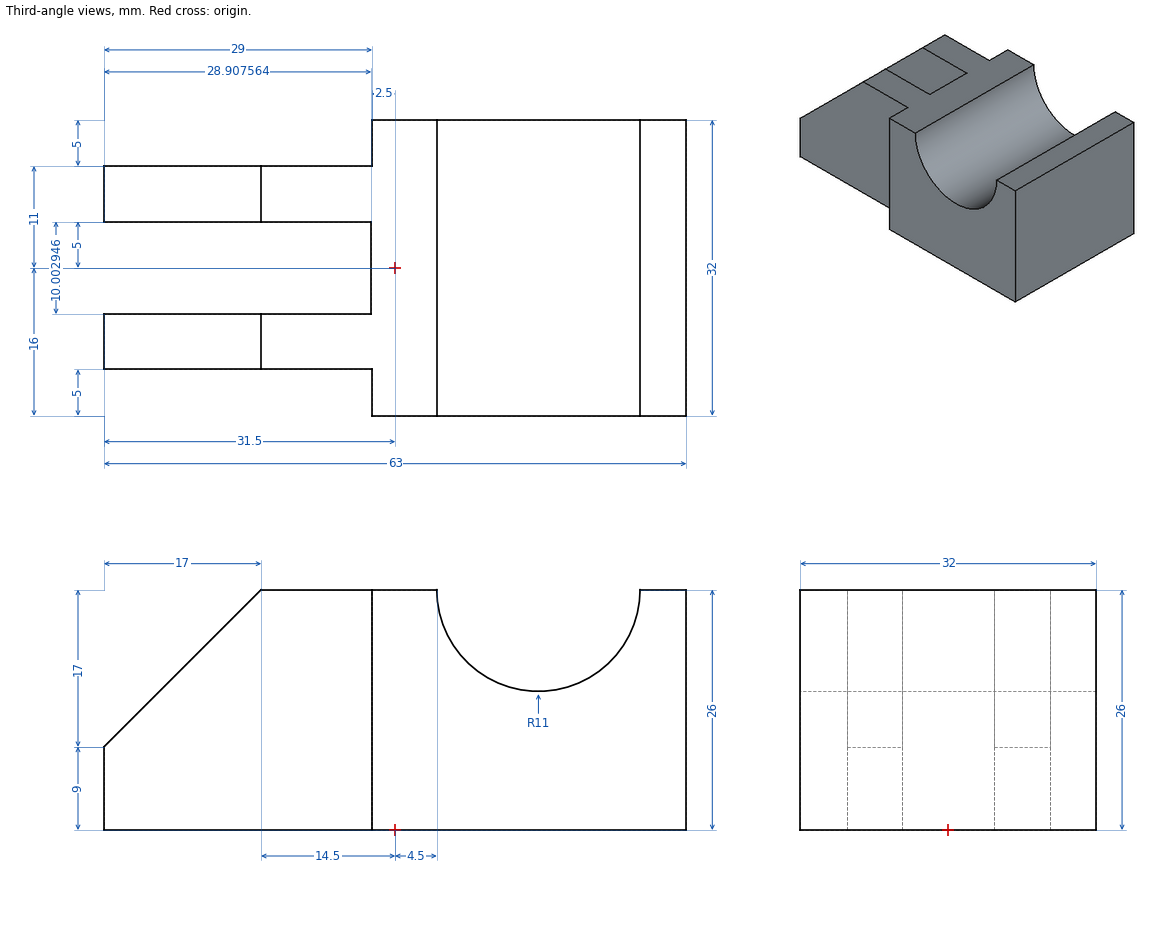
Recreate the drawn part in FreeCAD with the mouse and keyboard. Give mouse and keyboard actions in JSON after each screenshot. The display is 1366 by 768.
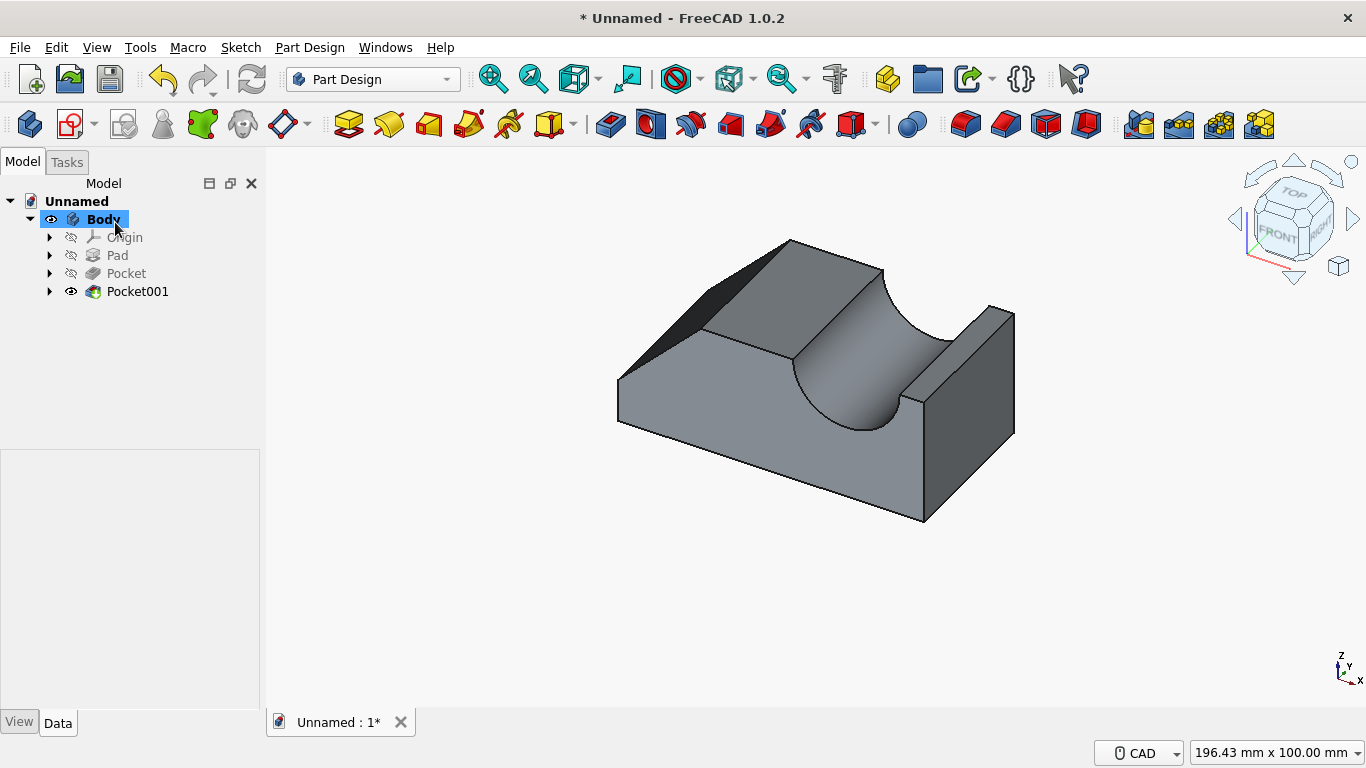
{"action": "key", "text": "5"}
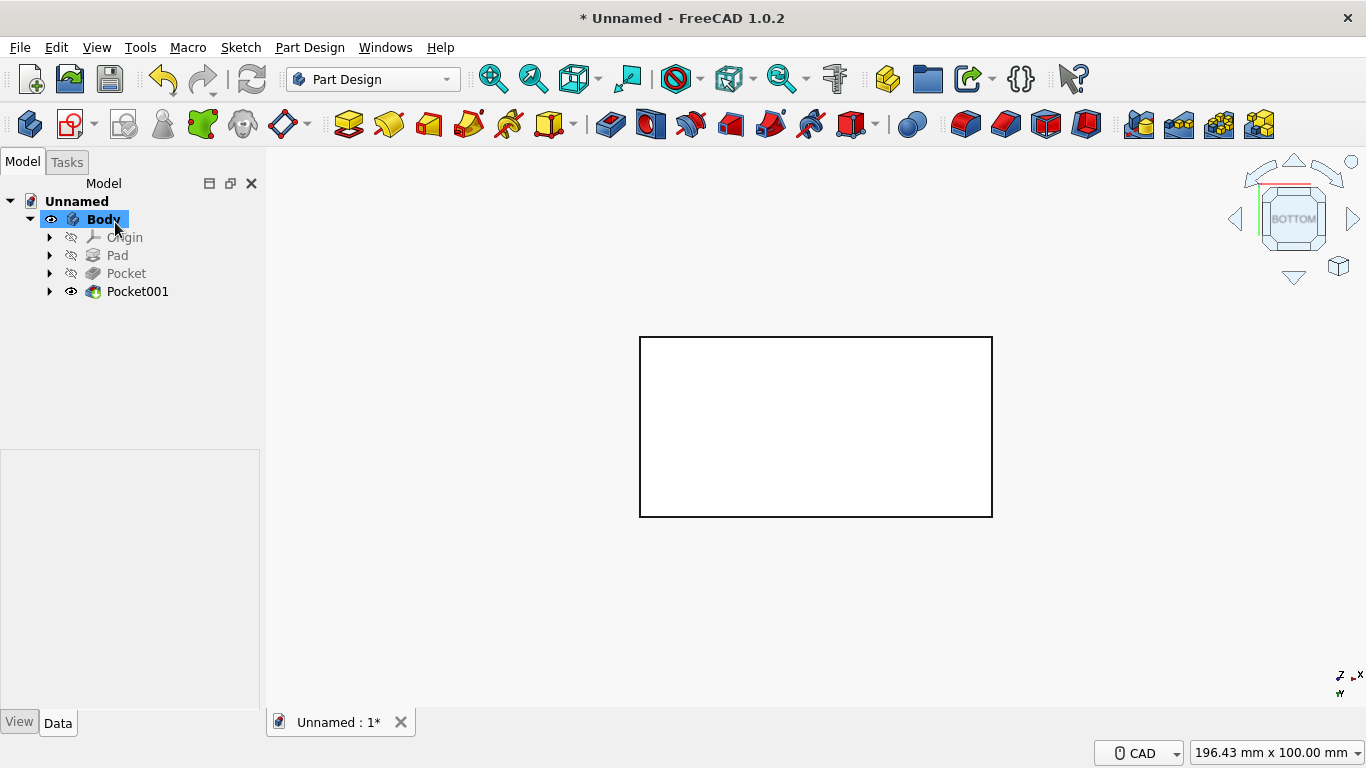
{"action": "left_click", "coordinate": [494, 80]}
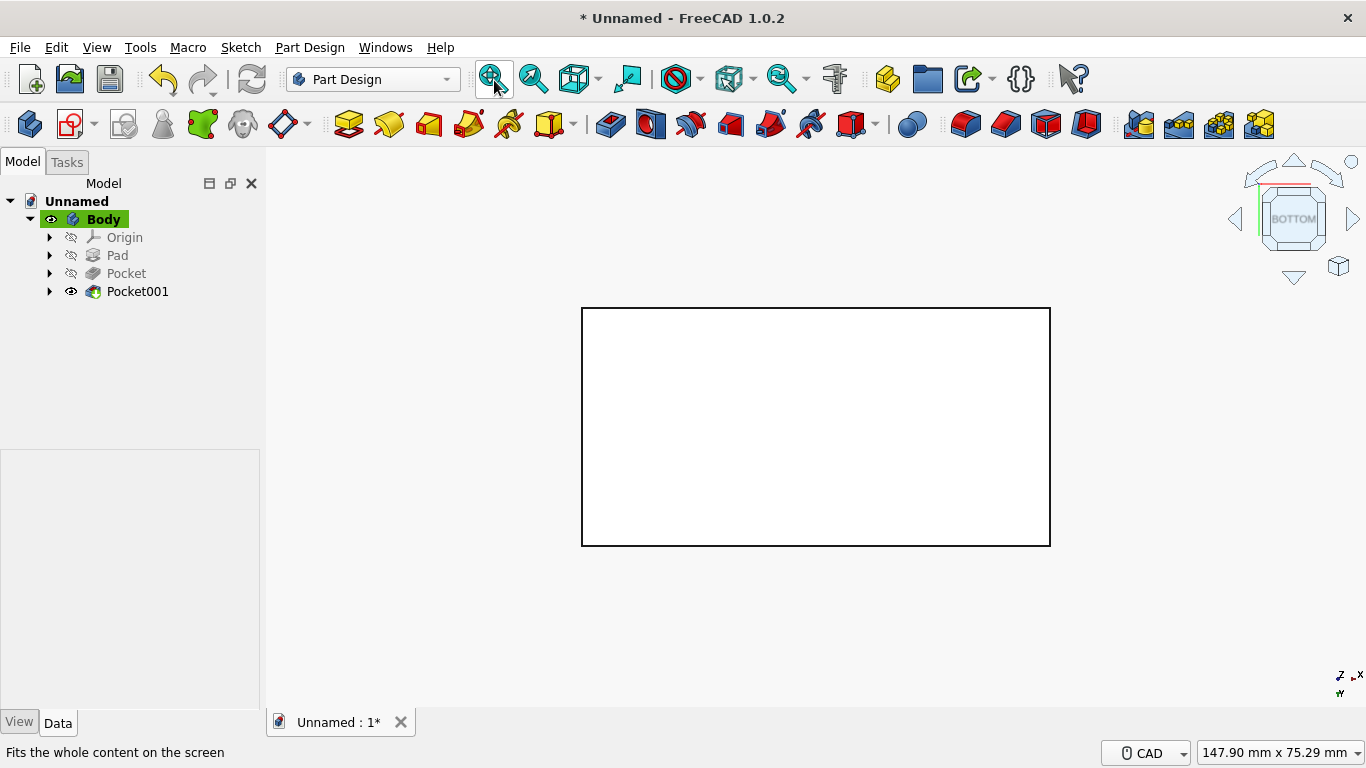
{"action": "left_click", "coordinate": [883, 426]}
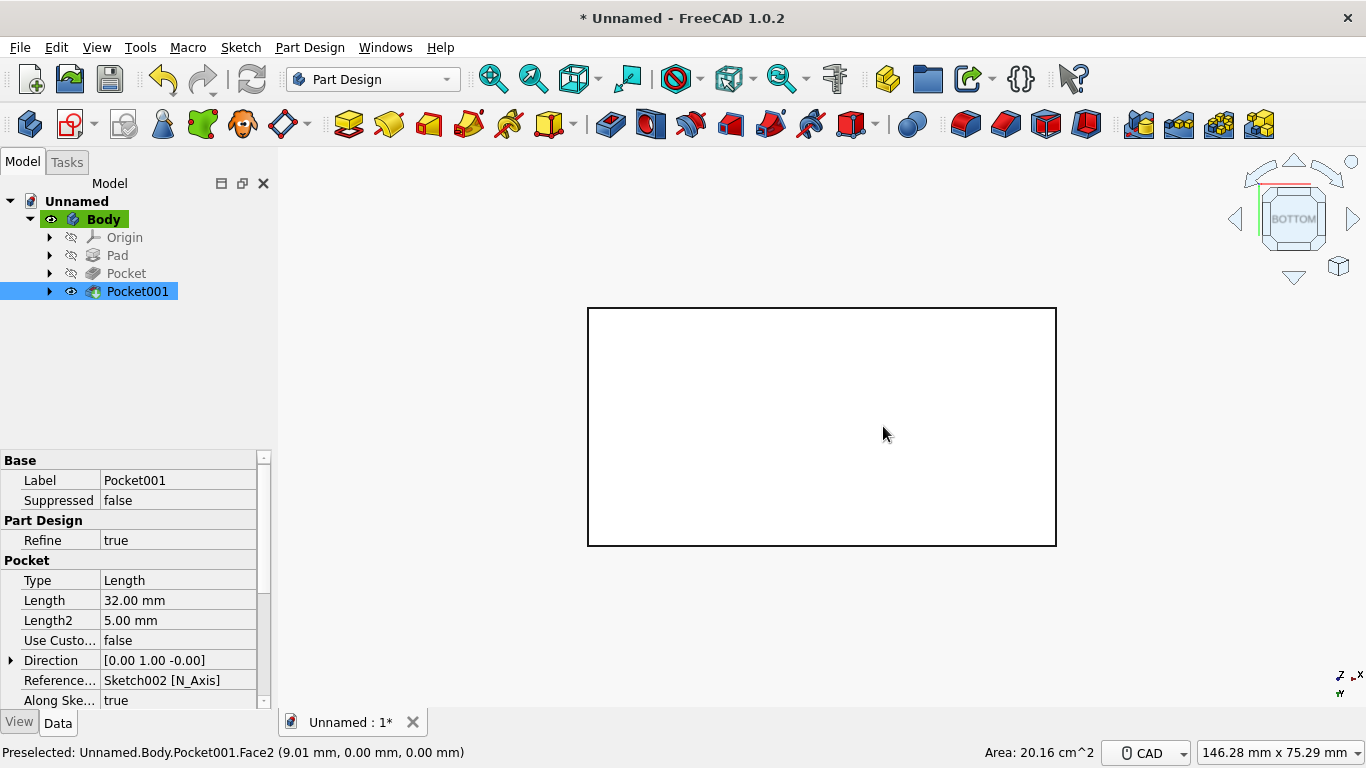
{"action": "left_click", "coordinate": [70, 124]}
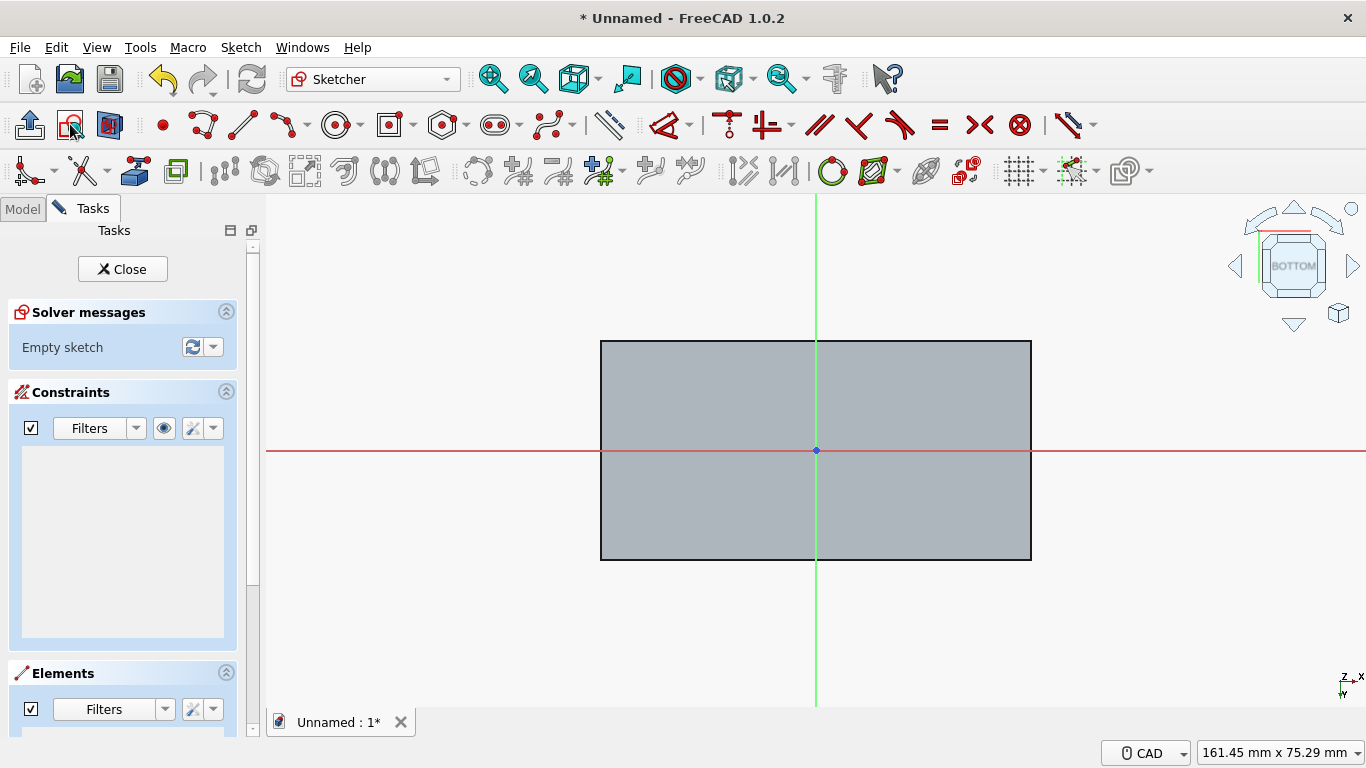
{"action": "scroll", "coordinate": [630, 451], "scroll_direction": "up", "scroll_amount": 2}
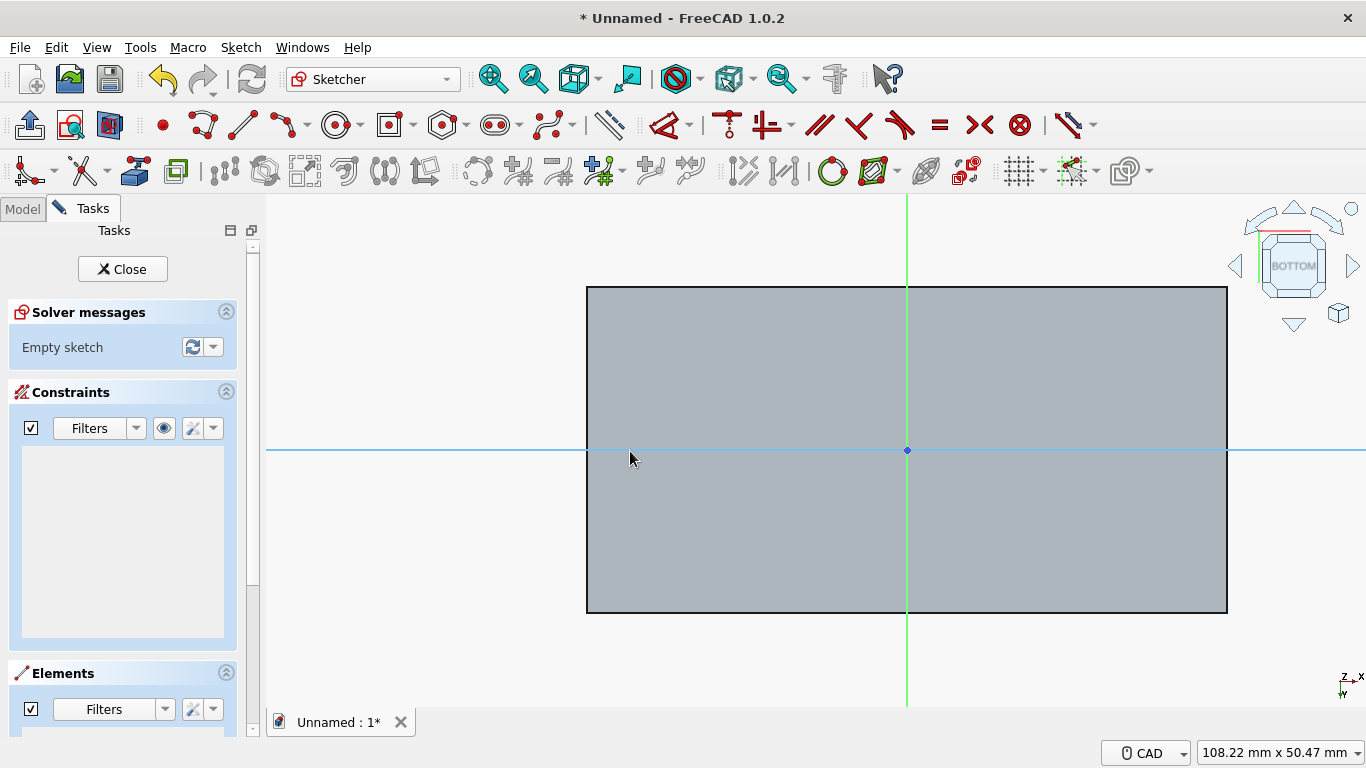
{"action": "left_click", "coordinate": [416, 126]}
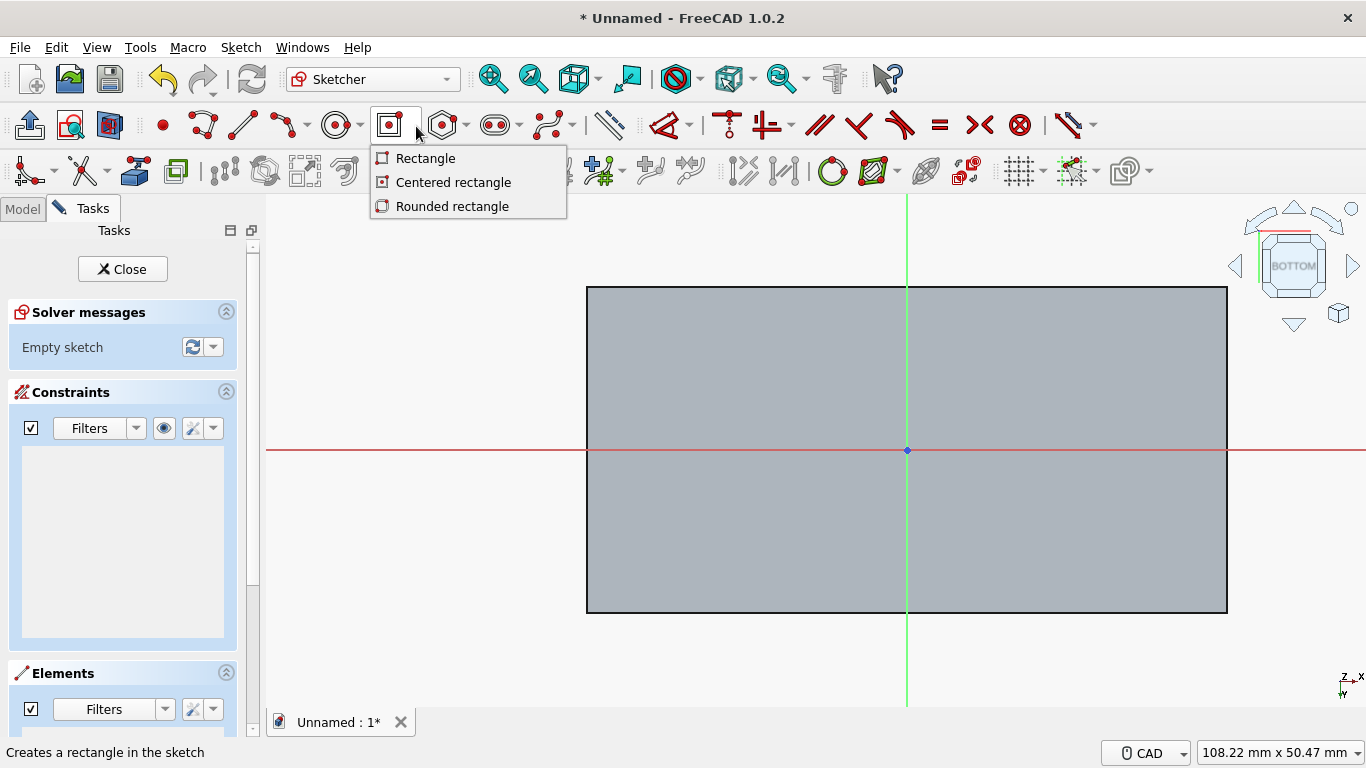
{"action": "left_click", "coordinate": [468, 158]}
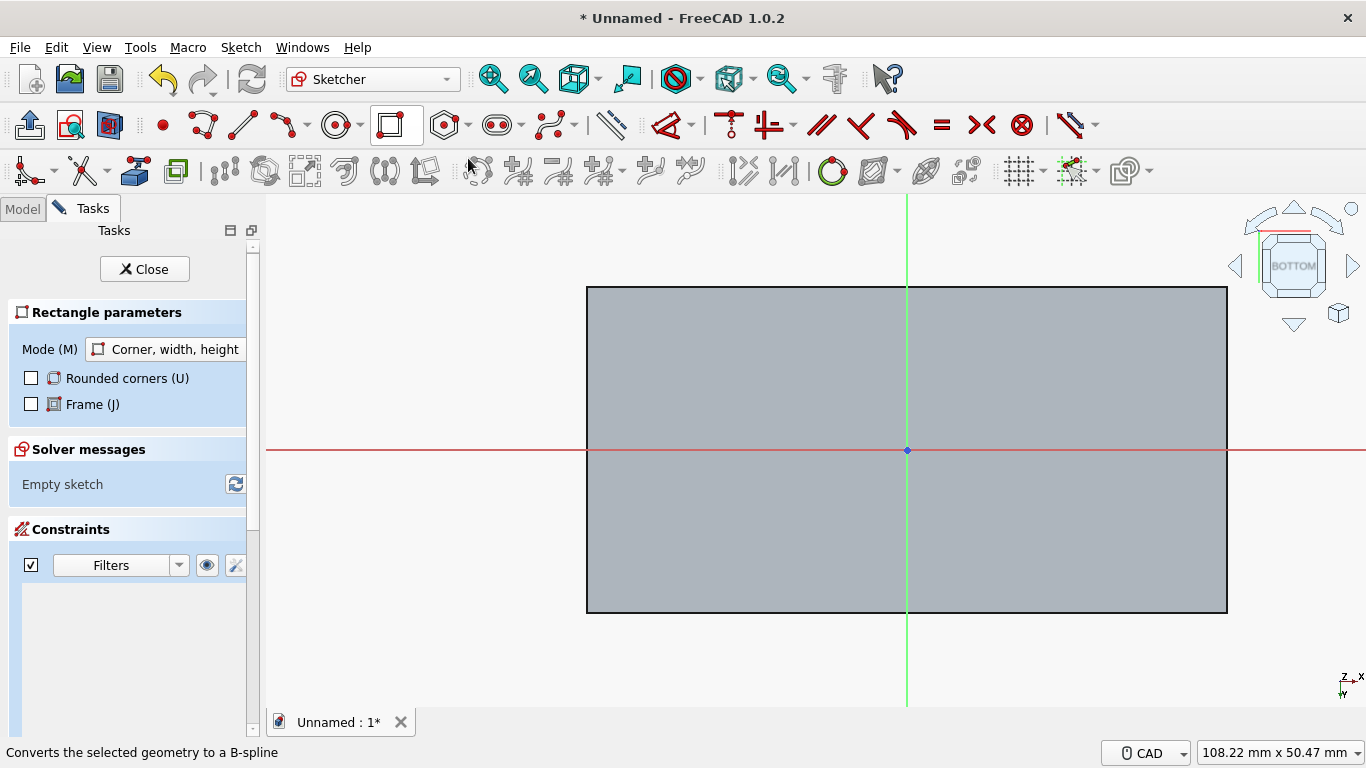
{"action": "left_click", "coordinate": [587, 562]}
{"action": "left_click", "coordinate": [882, 613]}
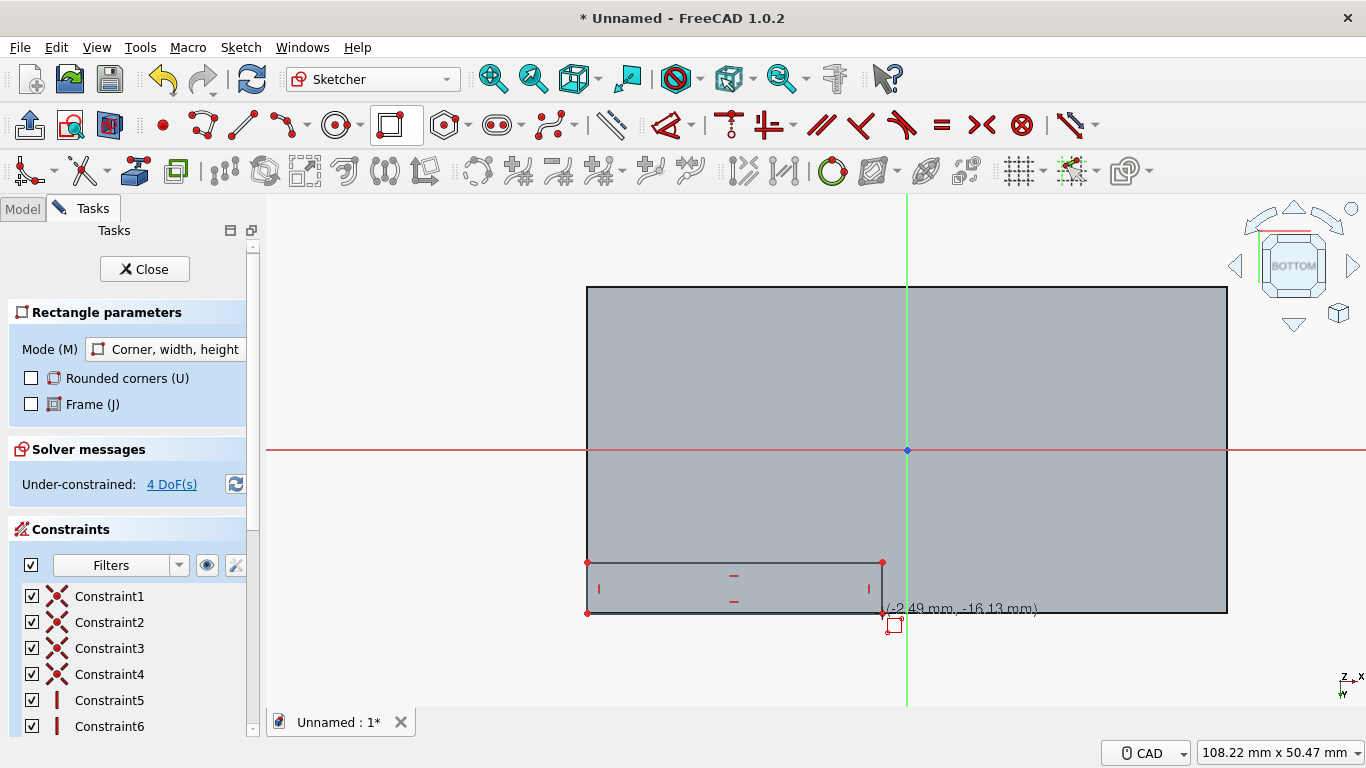
{"action": "left_click", "coordinate": [587, 287]}
{"action": "left_click", "coordinate": [882, 338]}
{"action": "key", "text": "Escape"}